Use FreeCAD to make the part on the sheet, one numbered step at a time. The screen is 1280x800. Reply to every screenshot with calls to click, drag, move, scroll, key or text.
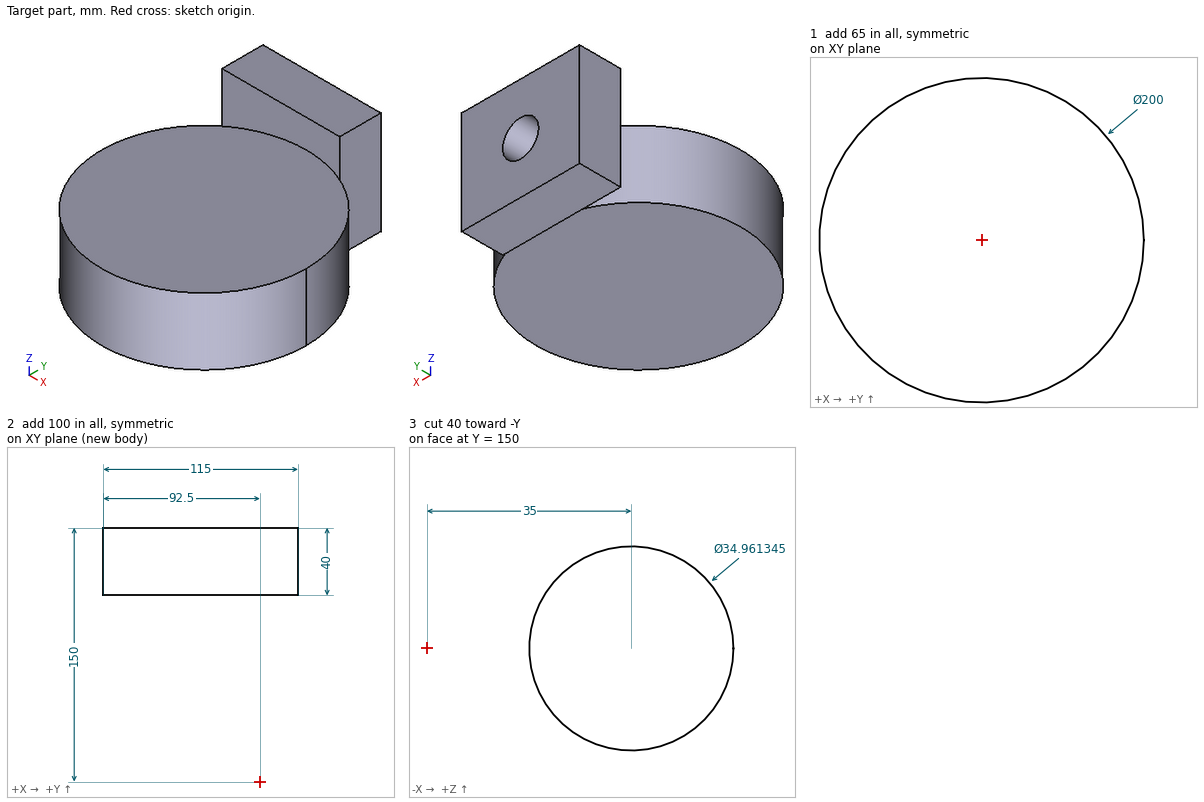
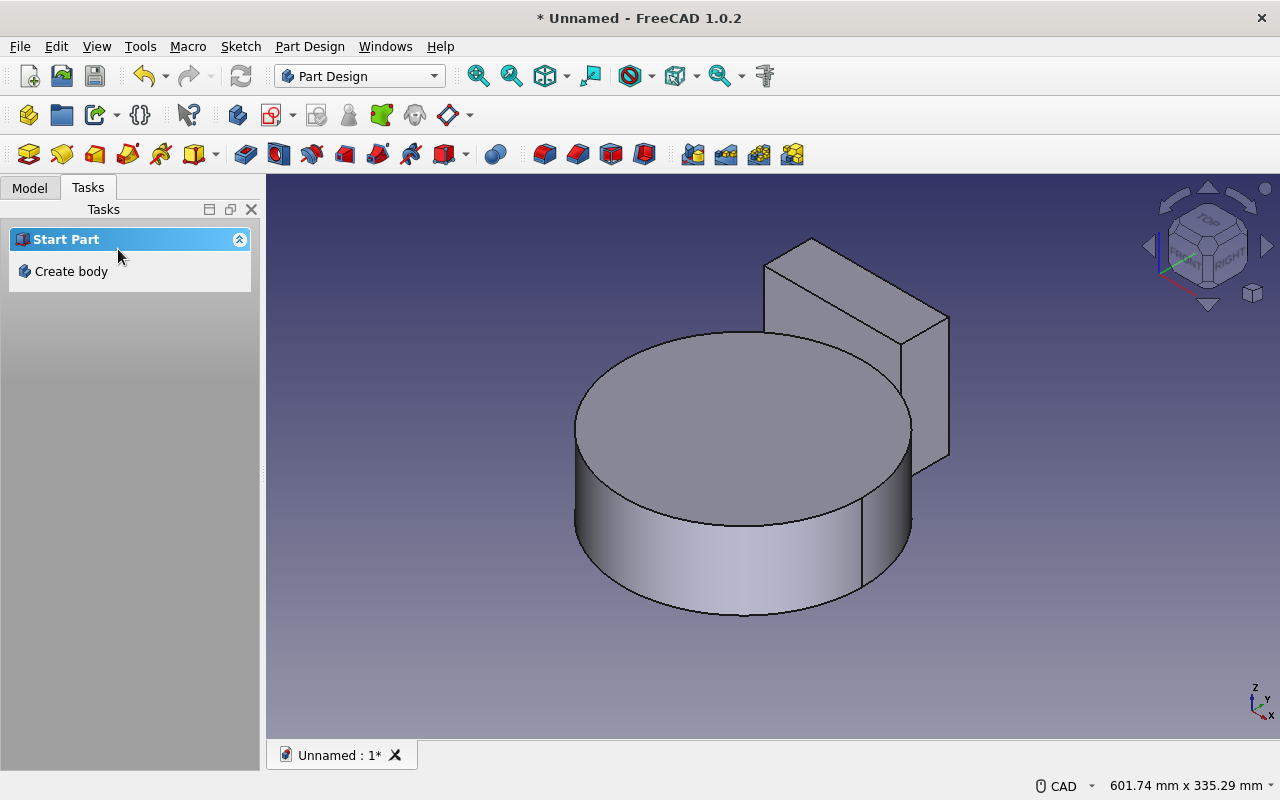
key(v)
key(f)